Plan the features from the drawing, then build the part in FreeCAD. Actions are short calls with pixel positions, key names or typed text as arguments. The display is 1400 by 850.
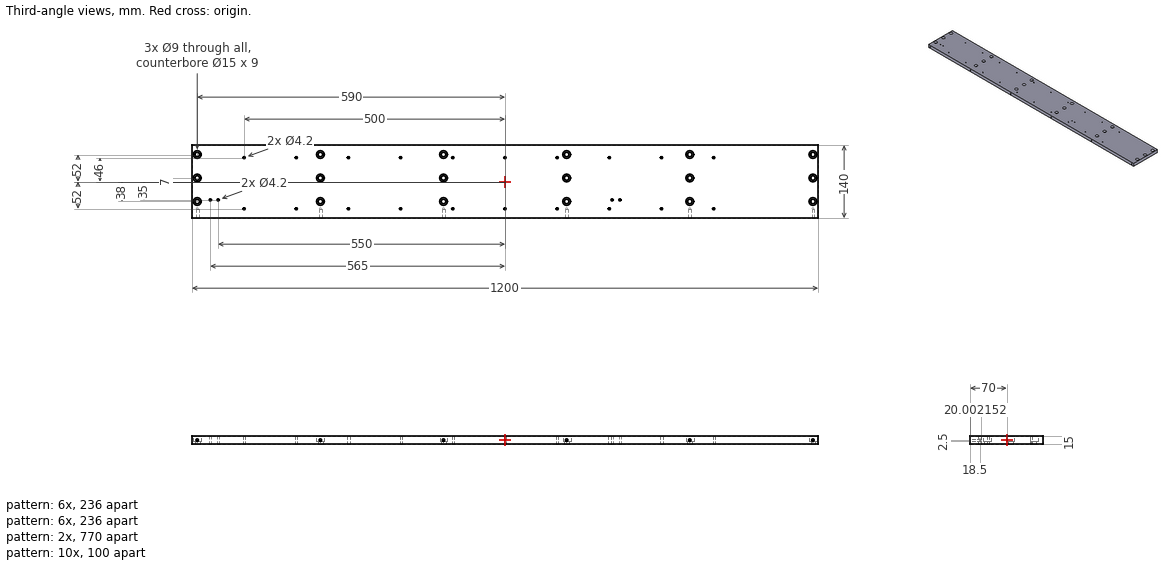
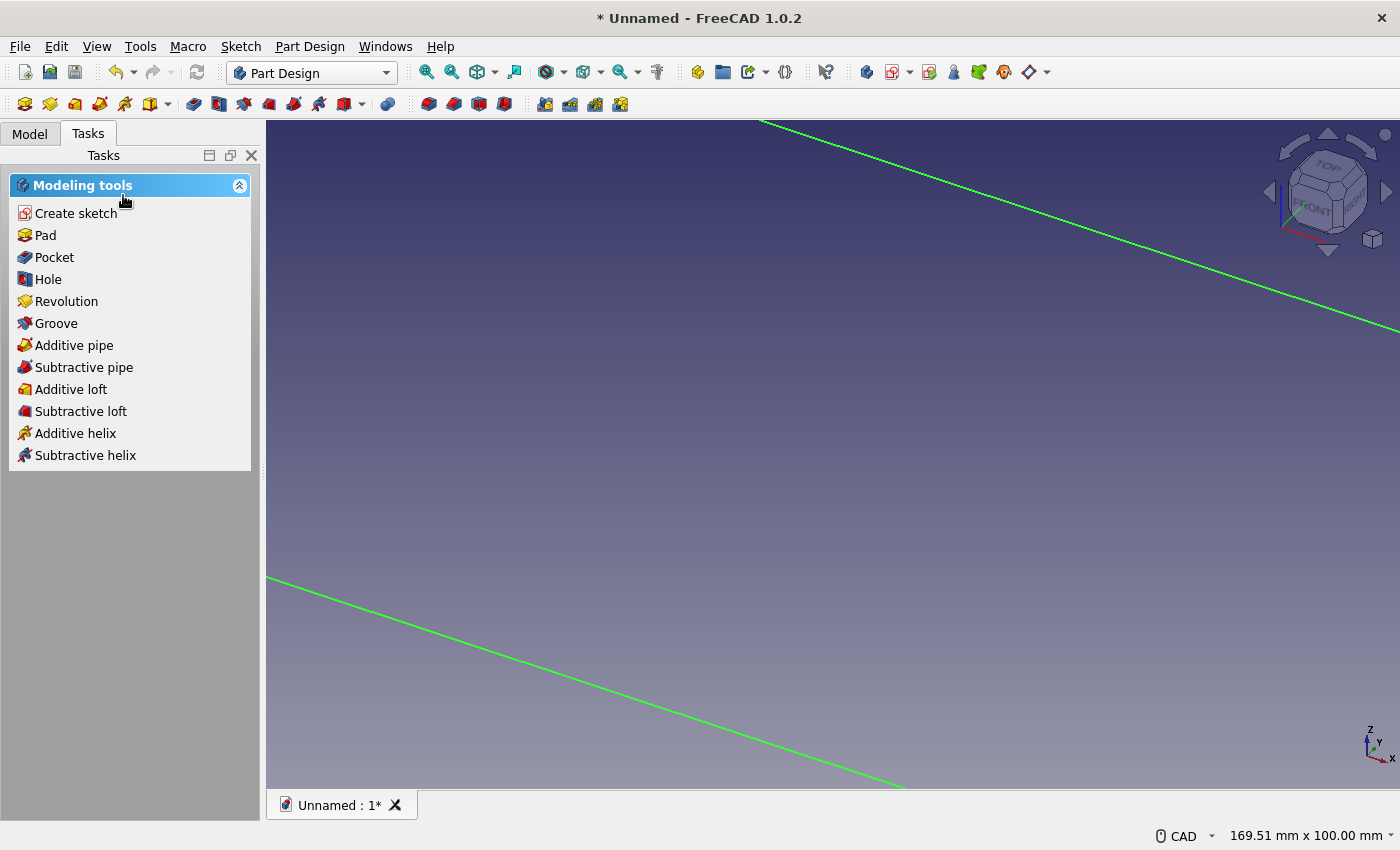
click(25, 104)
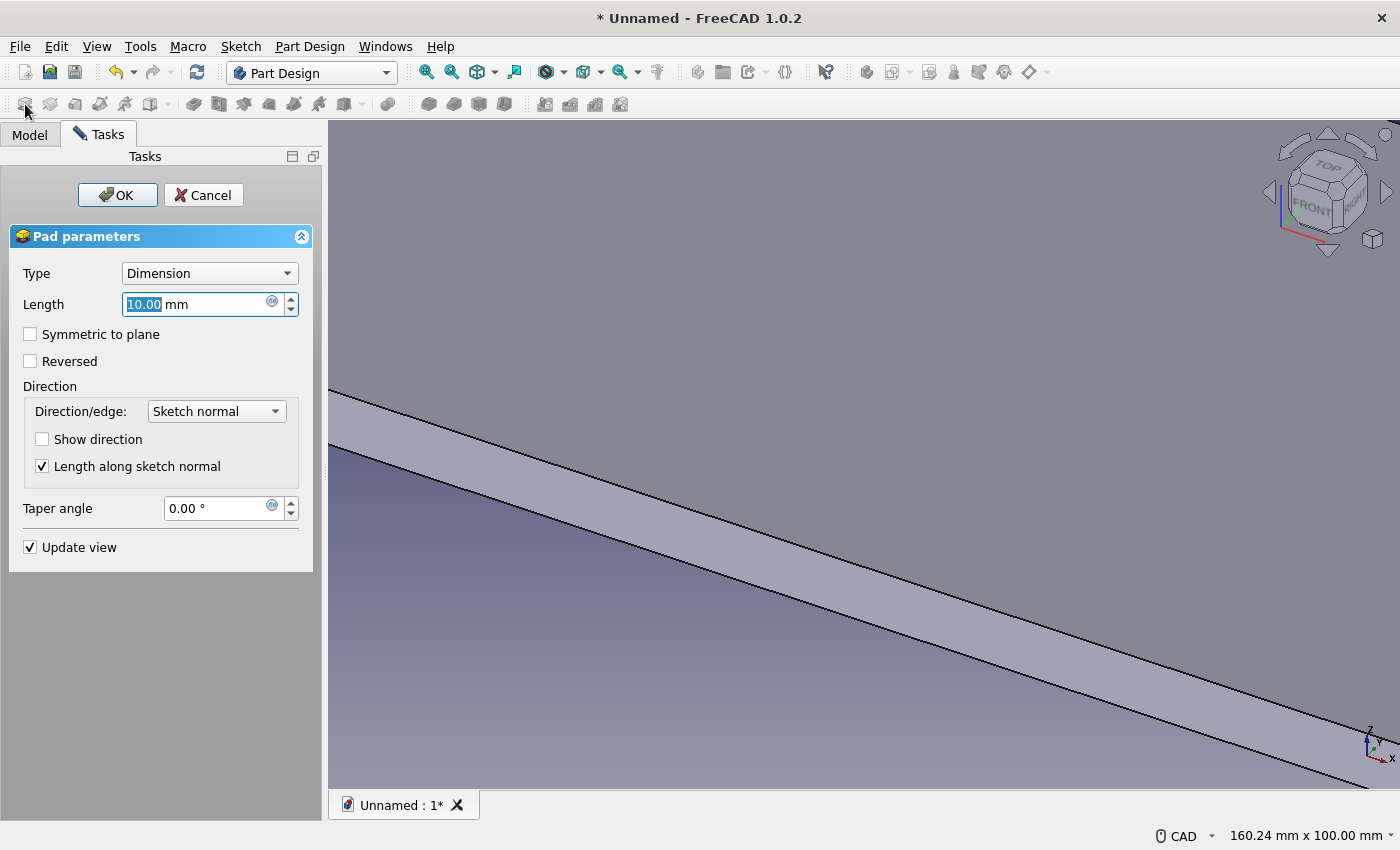
text(15)
key(Tab)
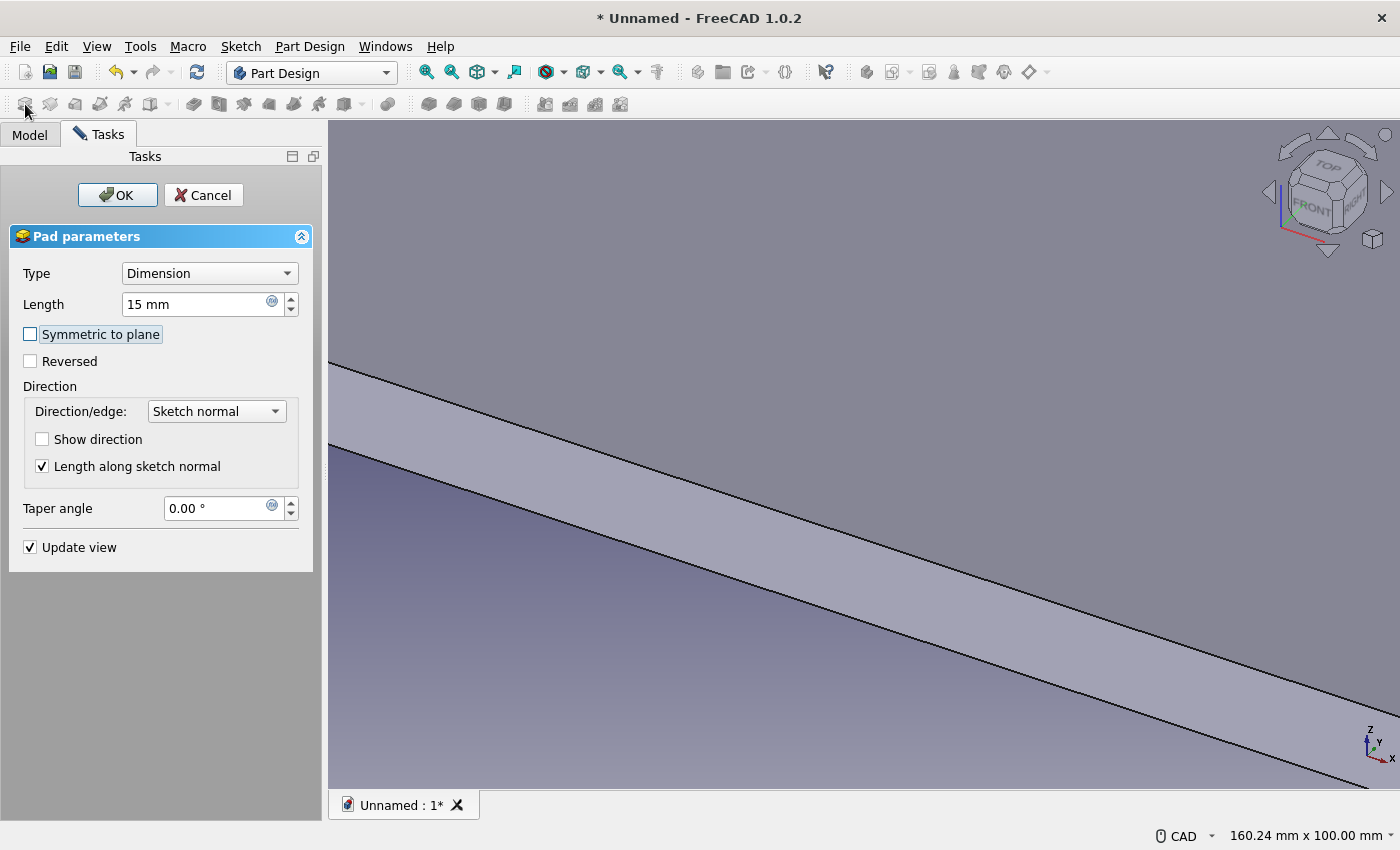
click(31, 334)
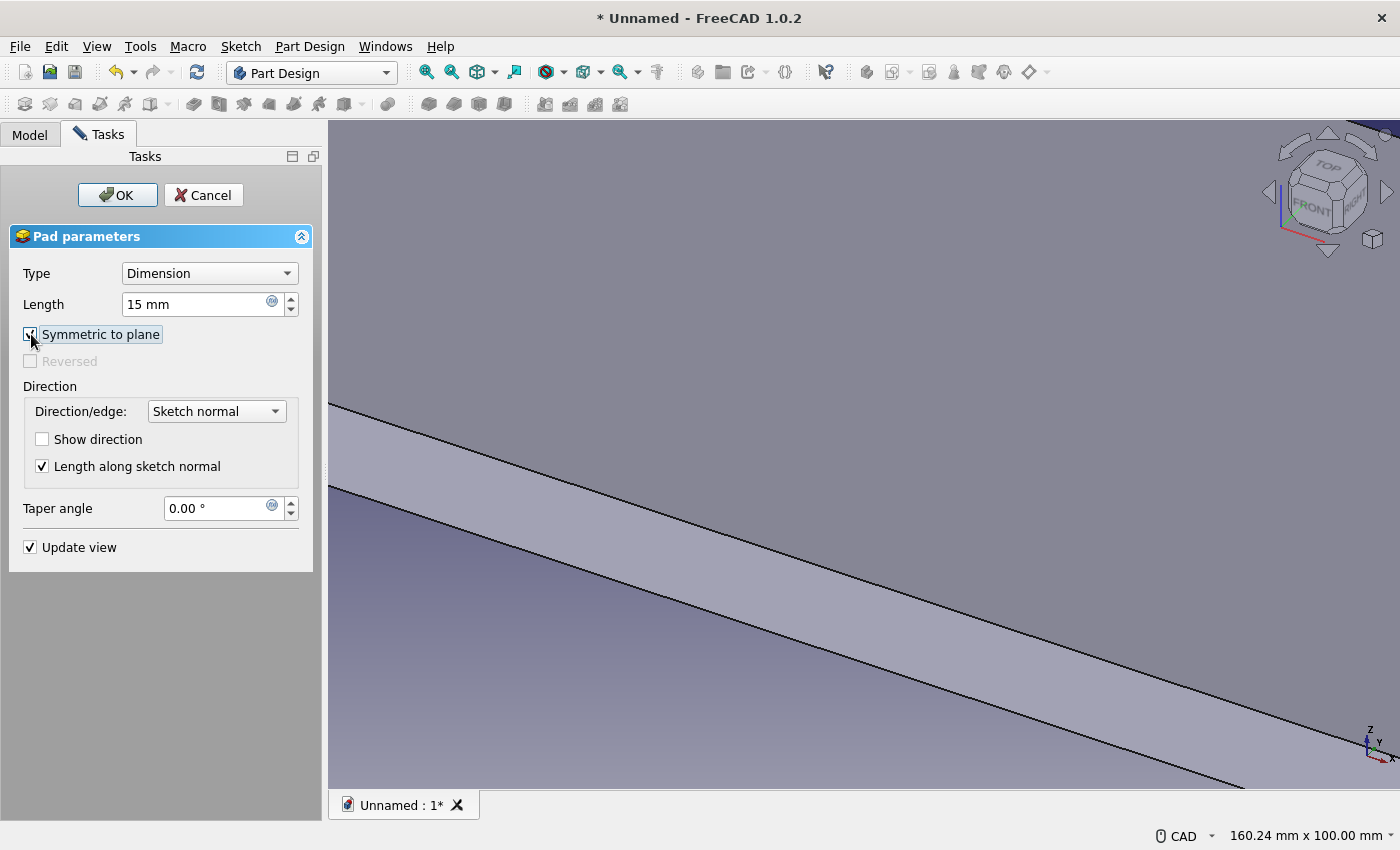
click(118, 195)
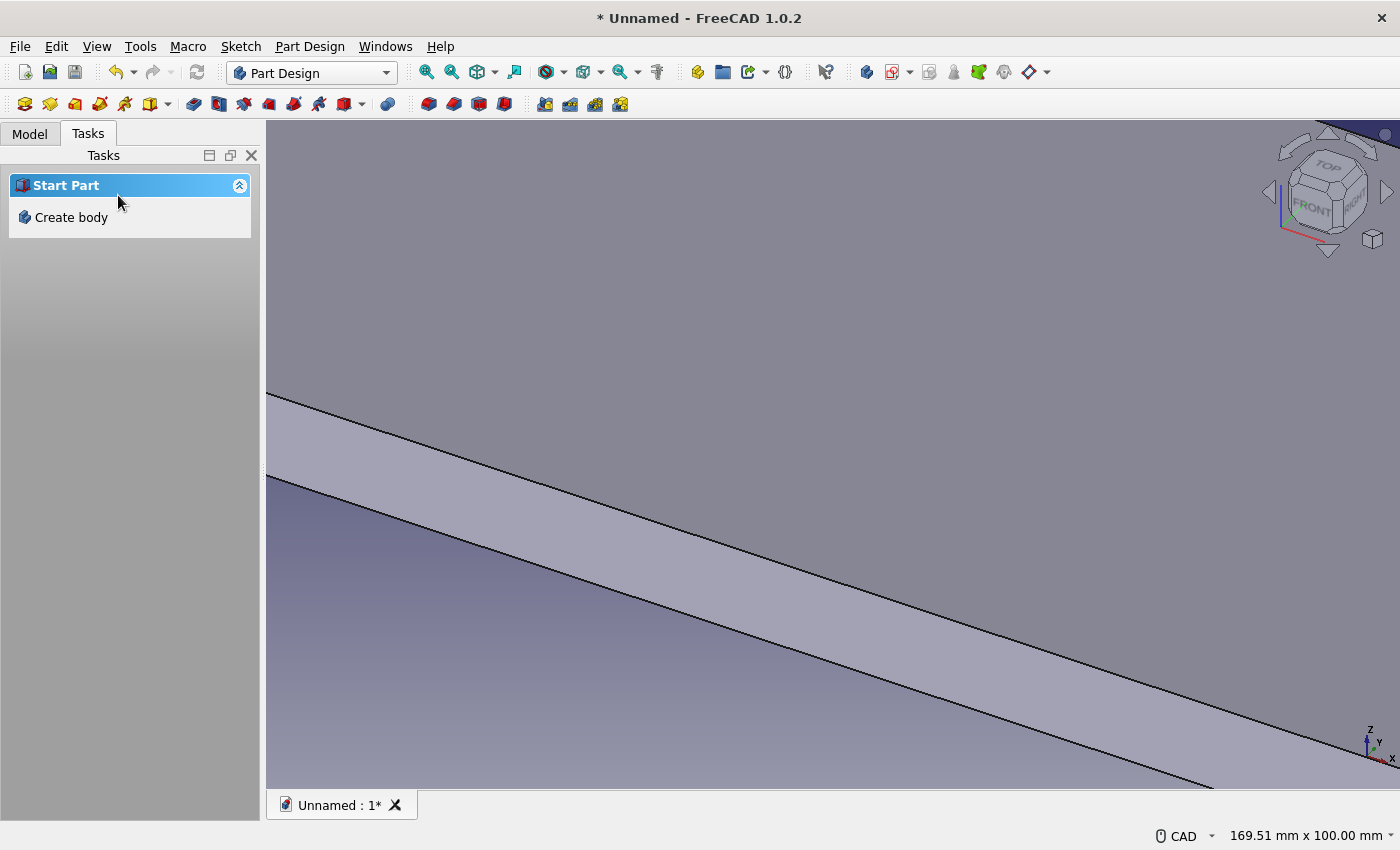
key(v)
key(f)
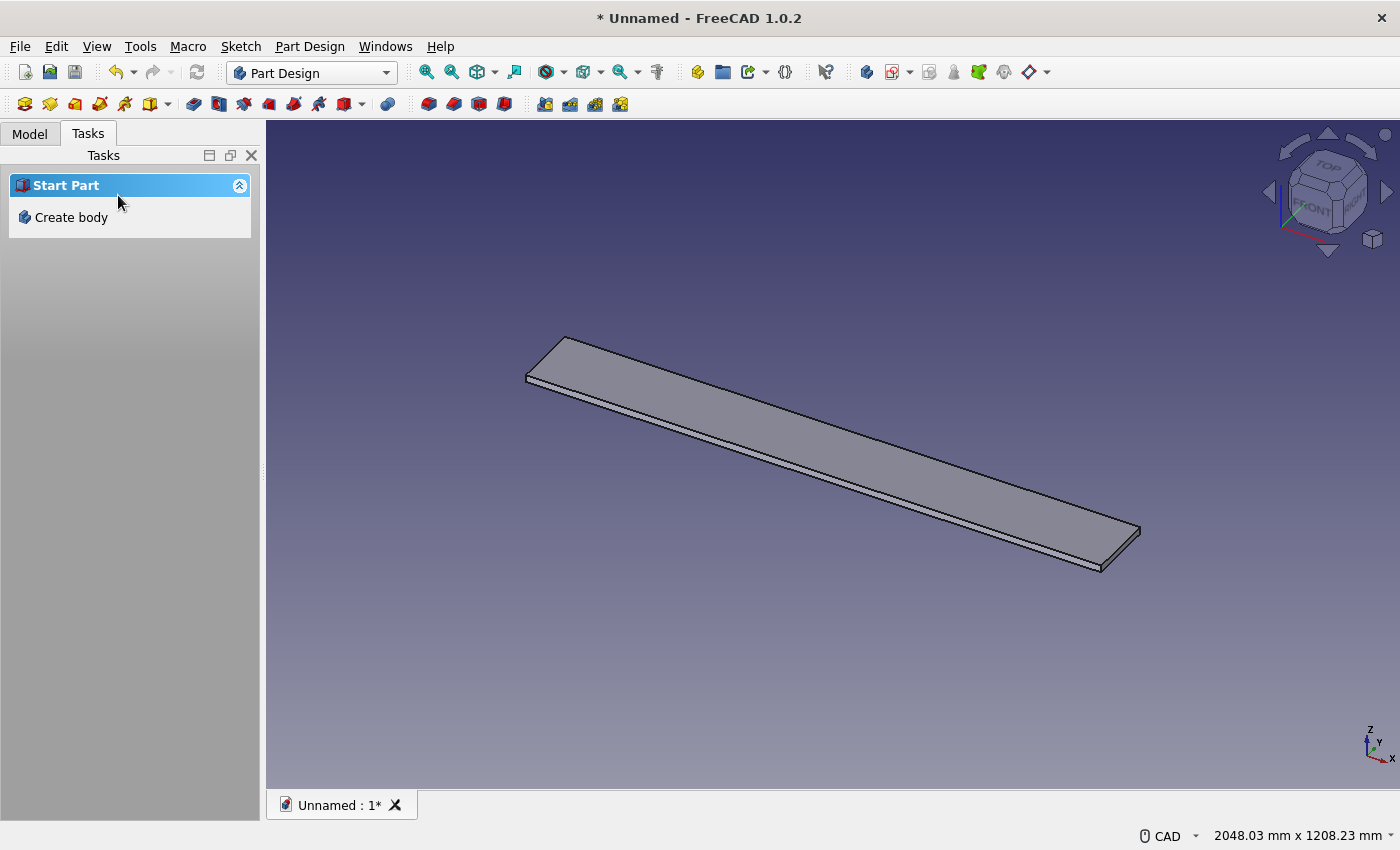
click(30, 134)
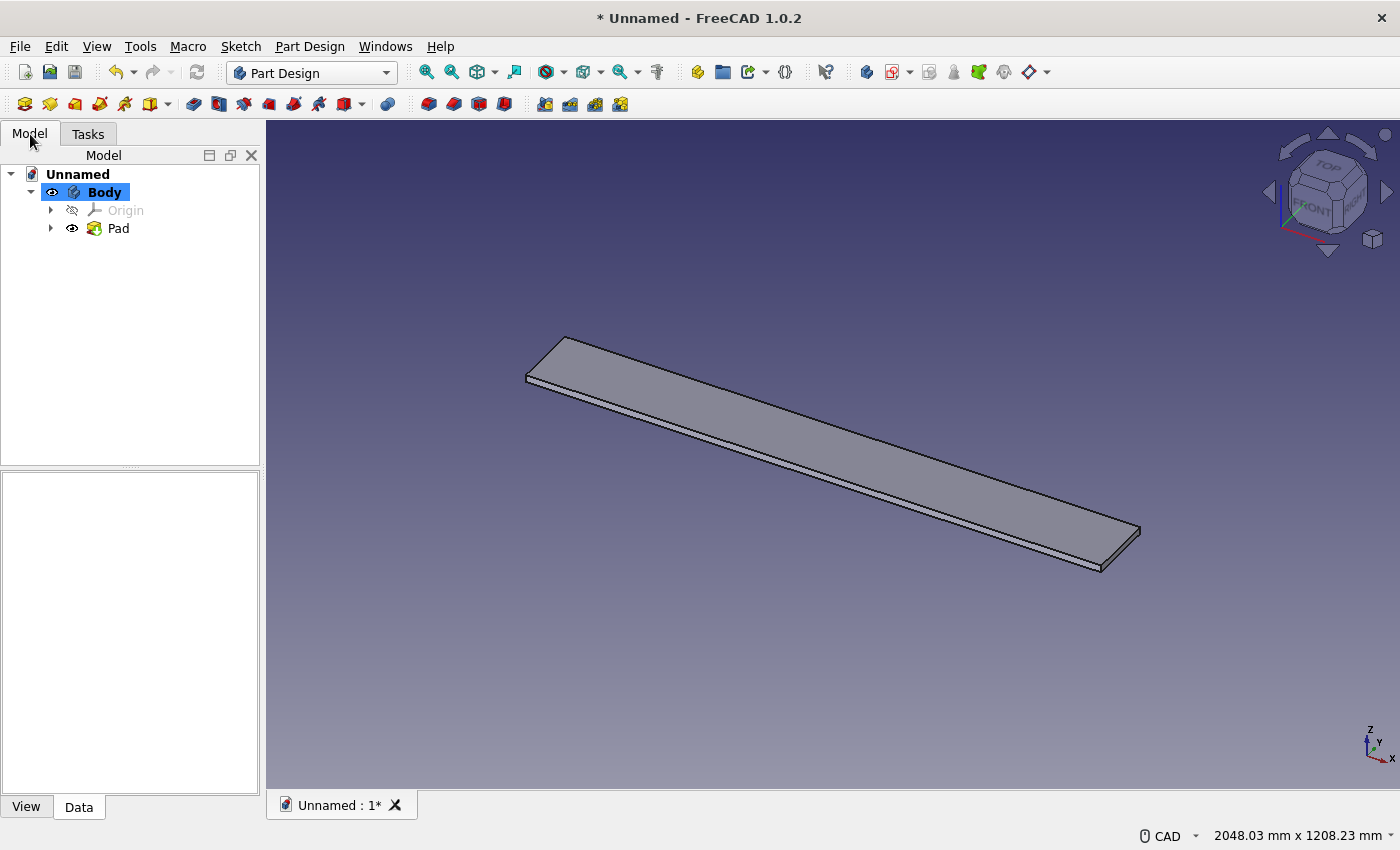
click(51, 210)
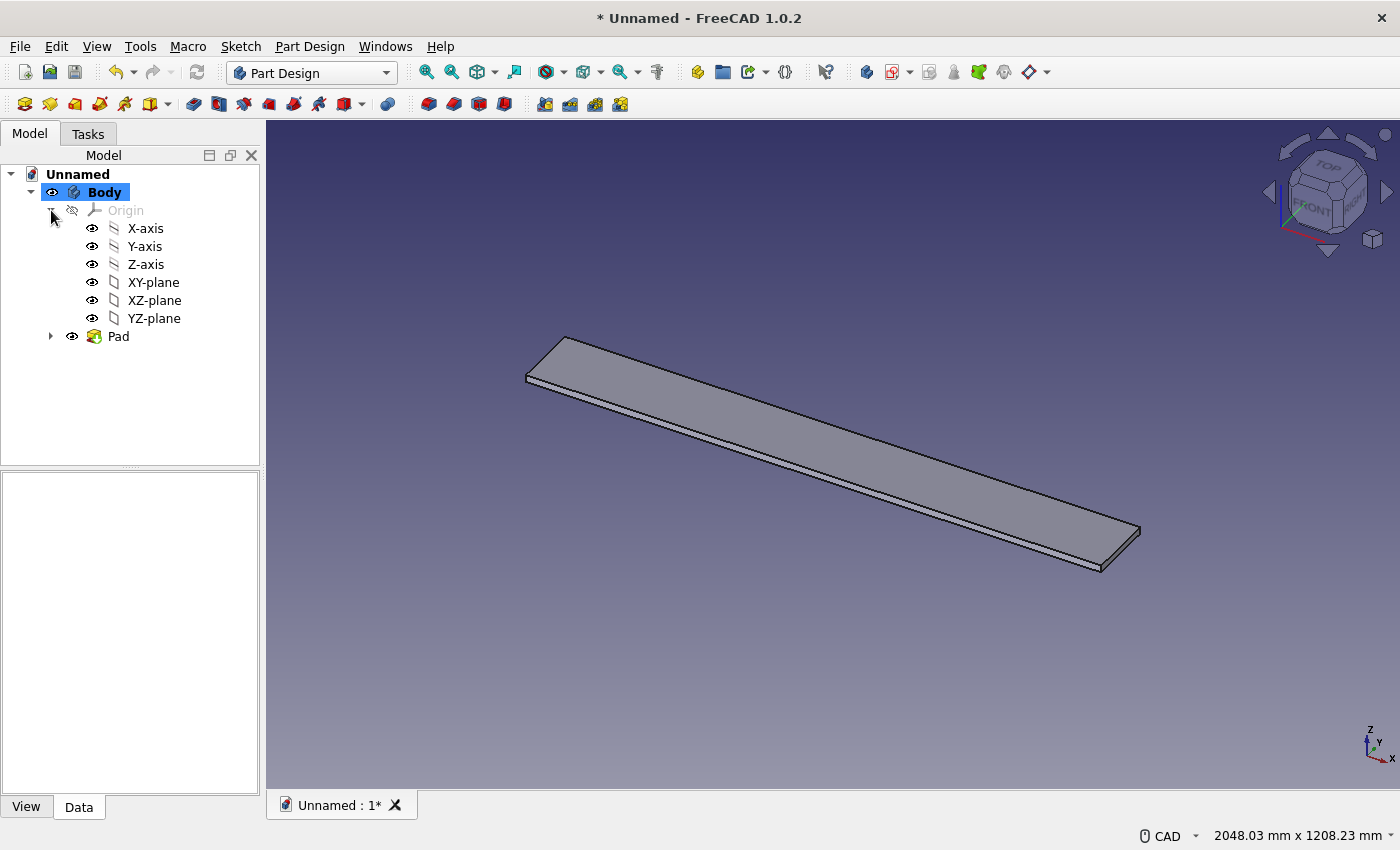
click(137, 318)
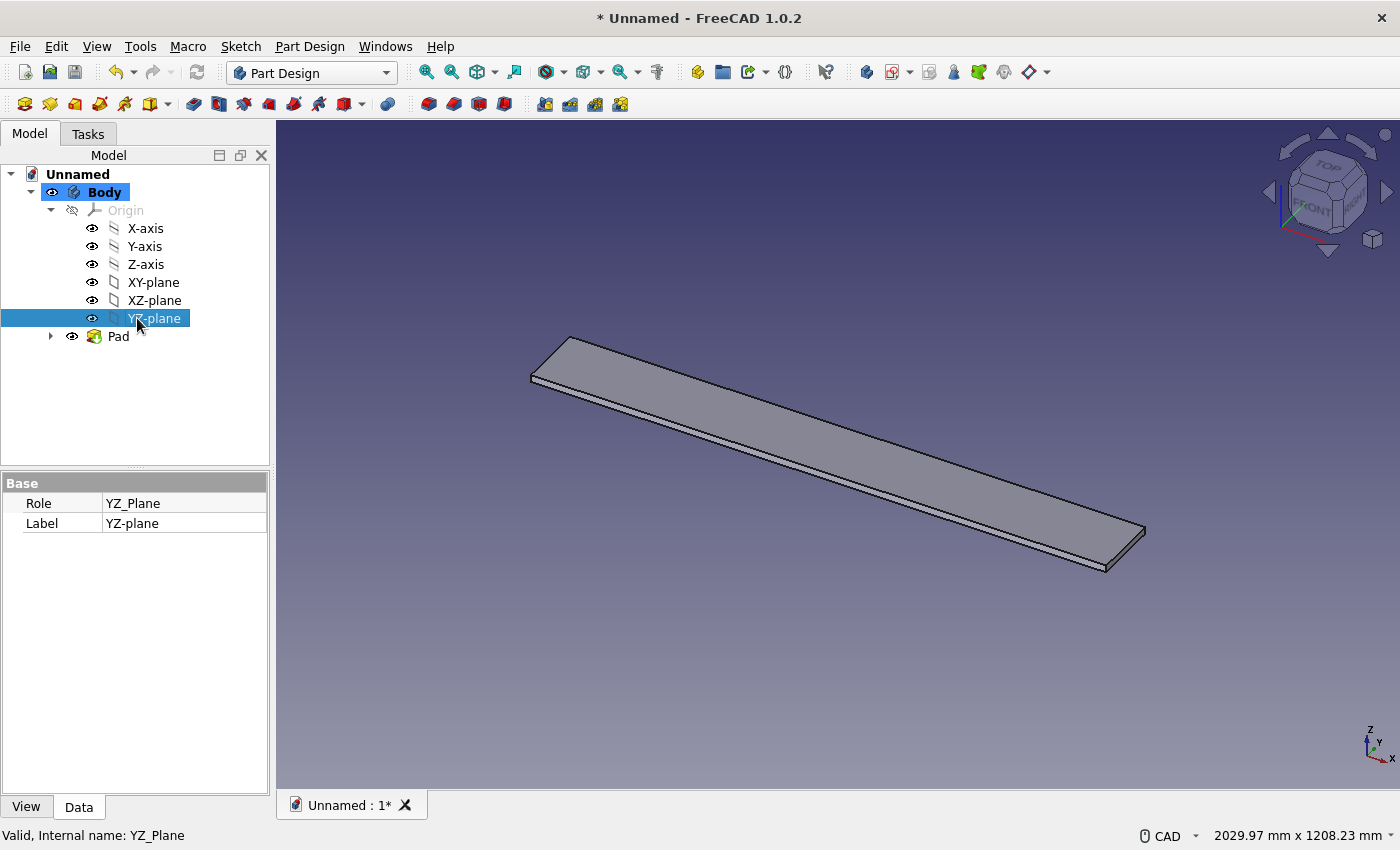
click(1028, 72)